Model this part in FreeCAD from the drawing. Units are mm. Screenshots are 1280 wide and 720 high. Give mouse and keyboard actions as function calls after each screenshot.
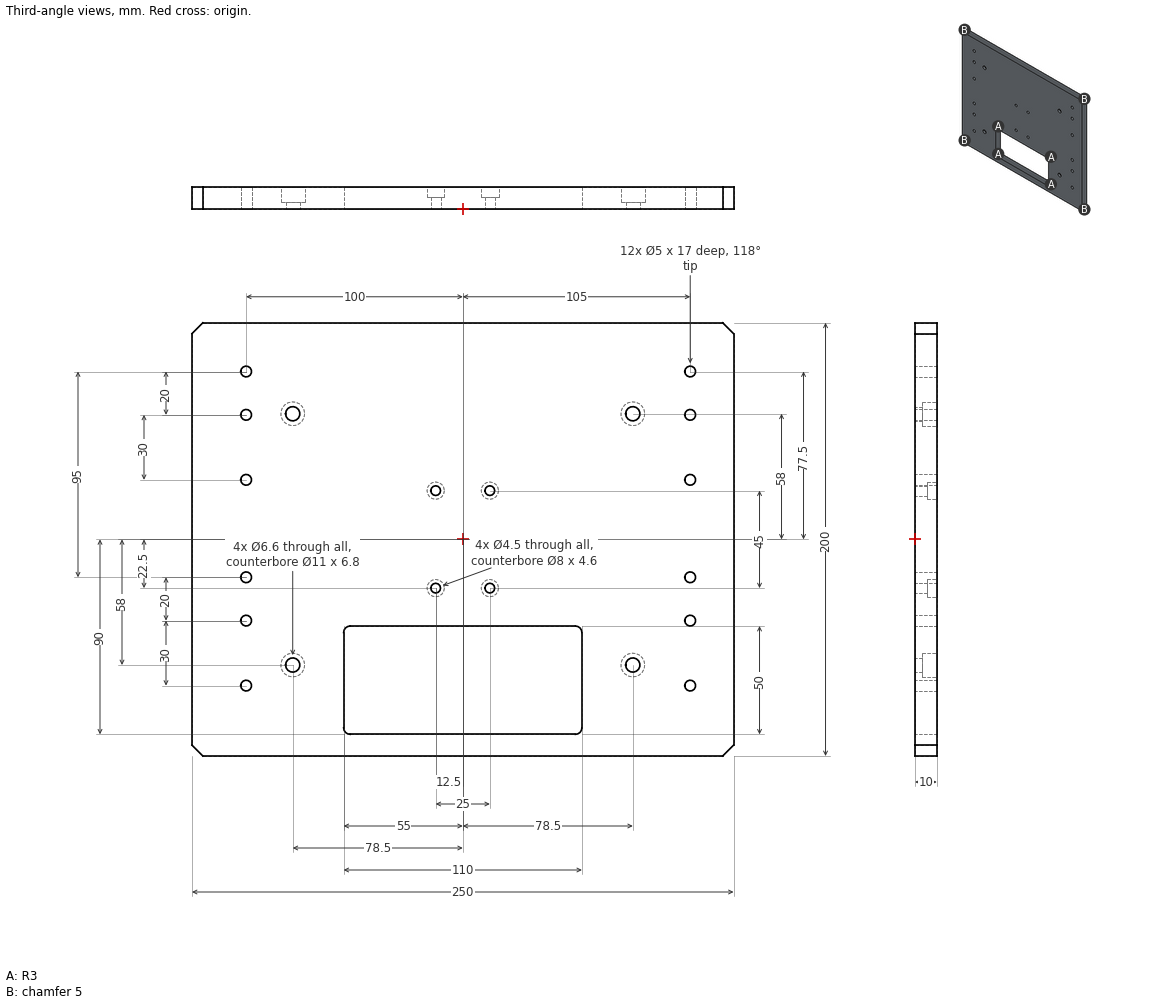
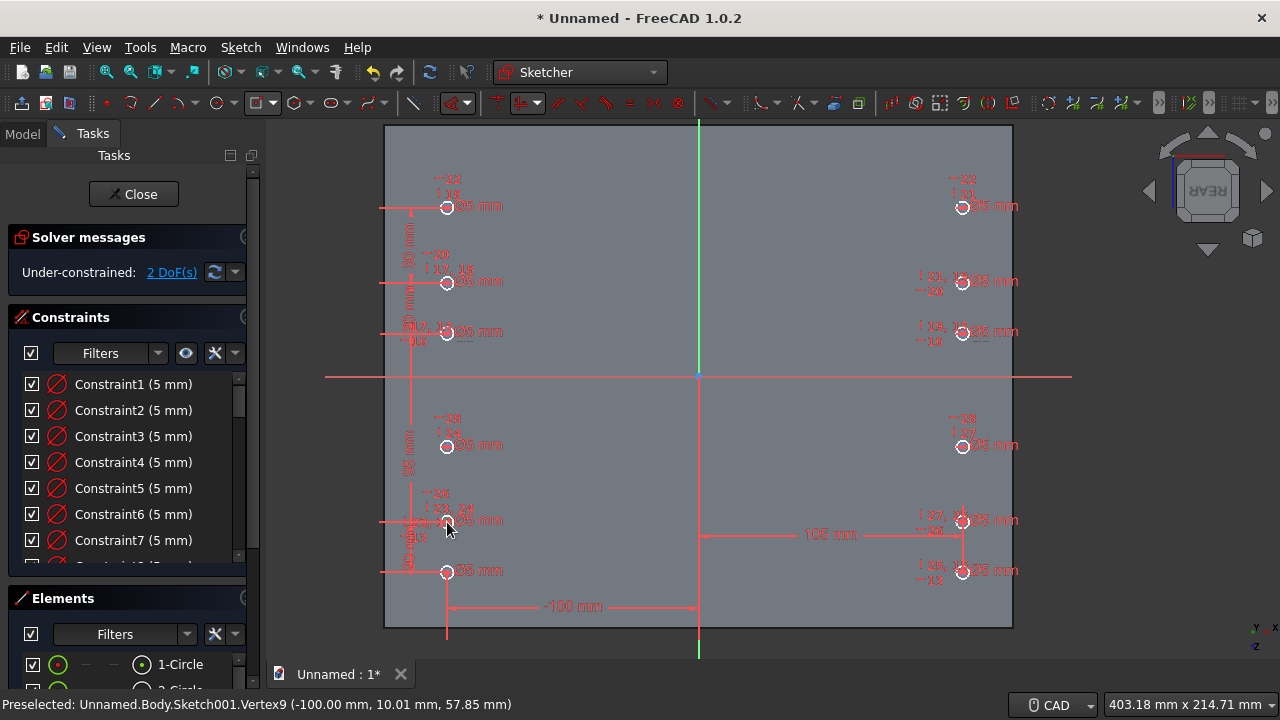
click(447, 447)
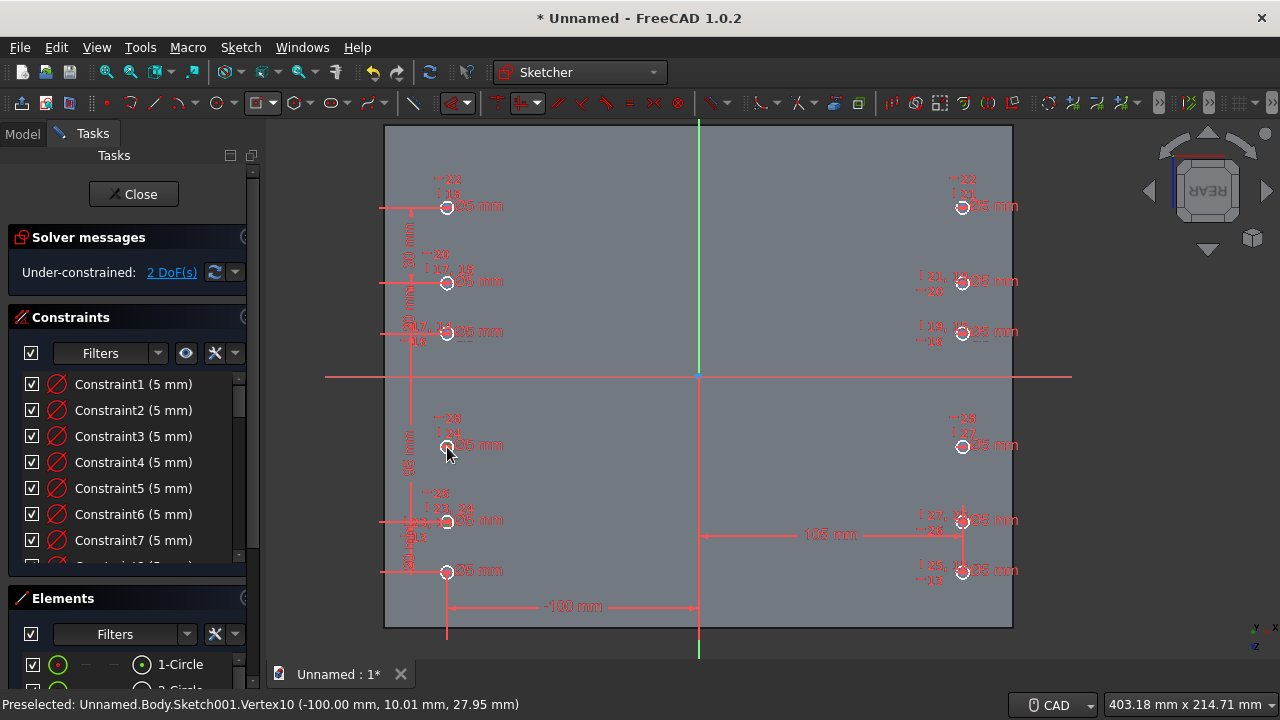
click(470, 104)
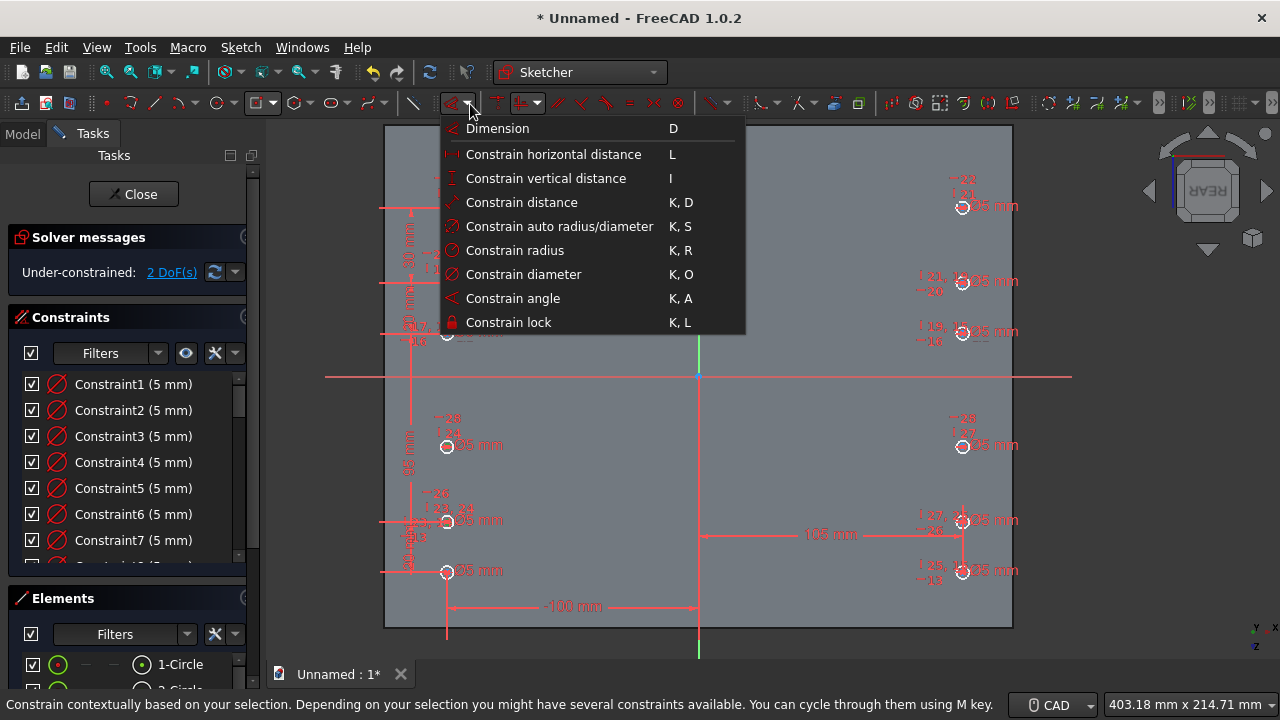
click(593, 178)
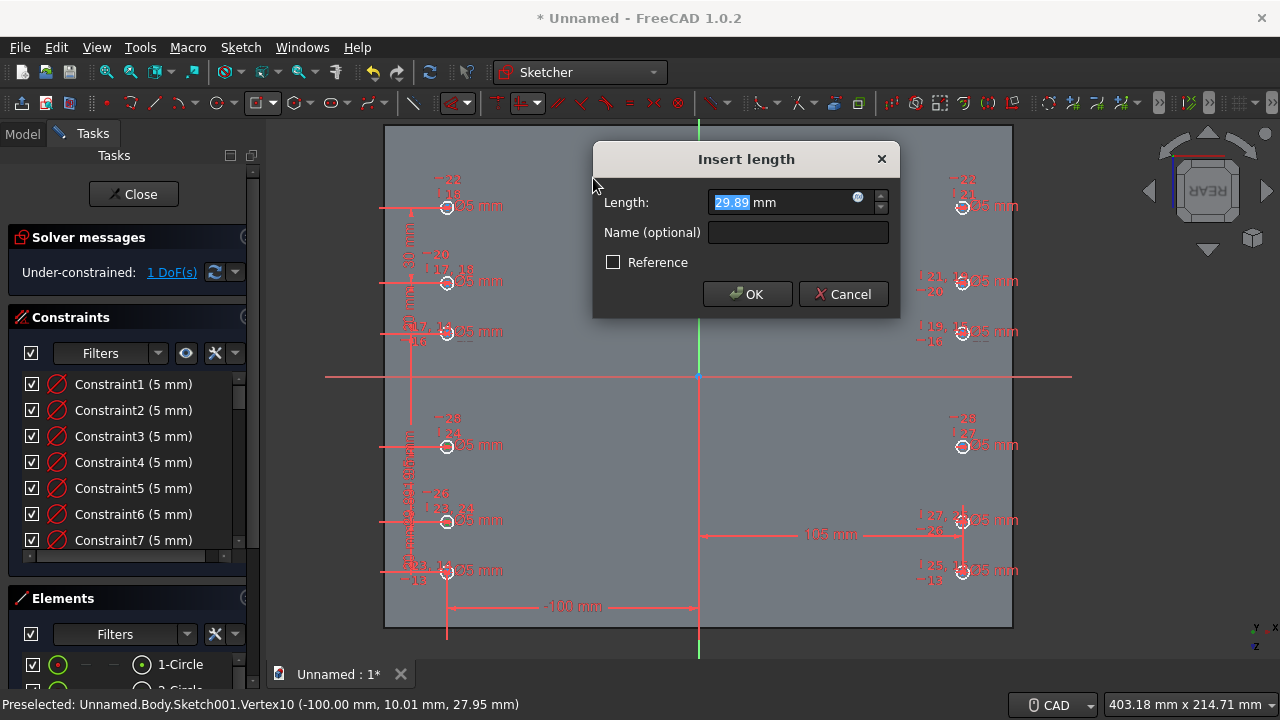
text(30)
key(Return)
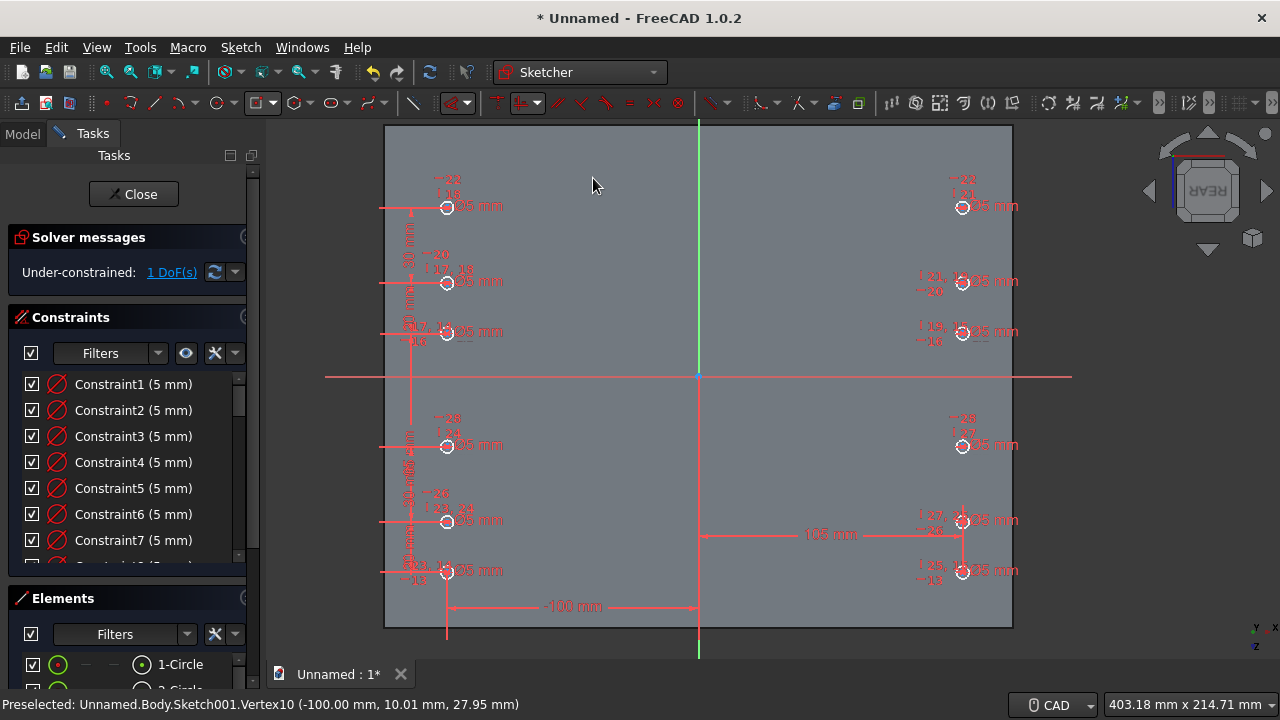
click(963, 572)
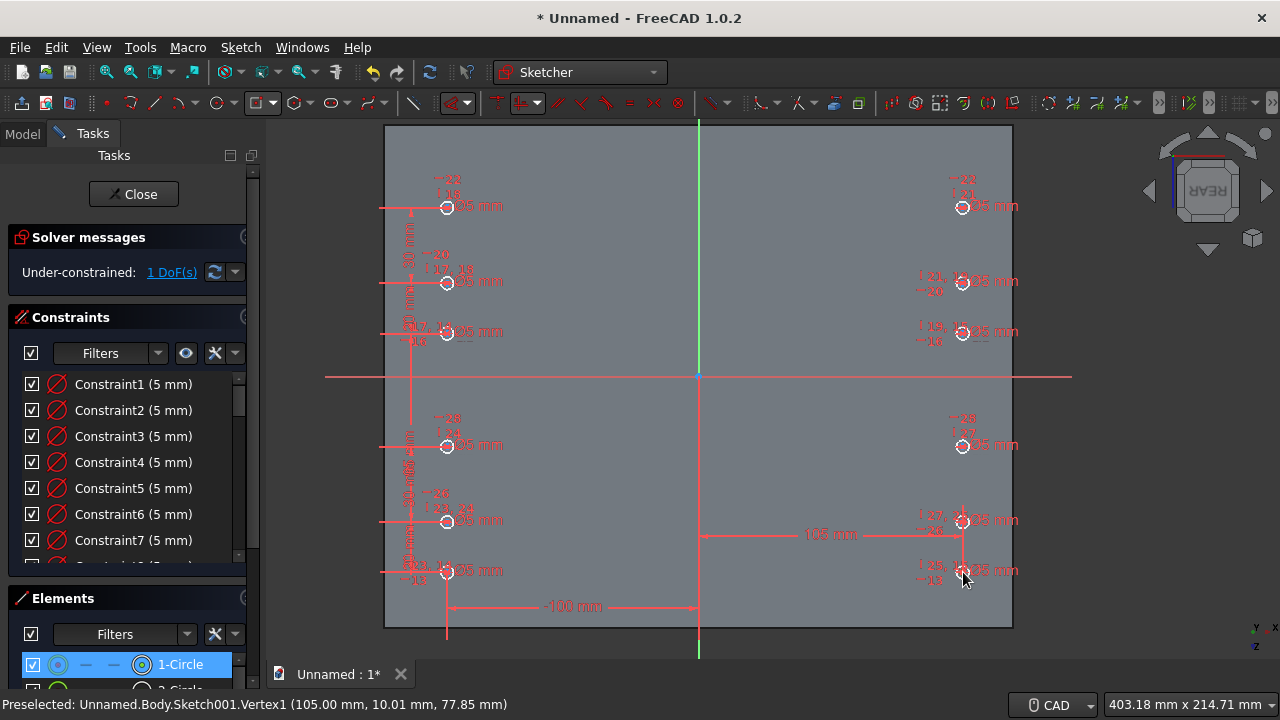
key(i)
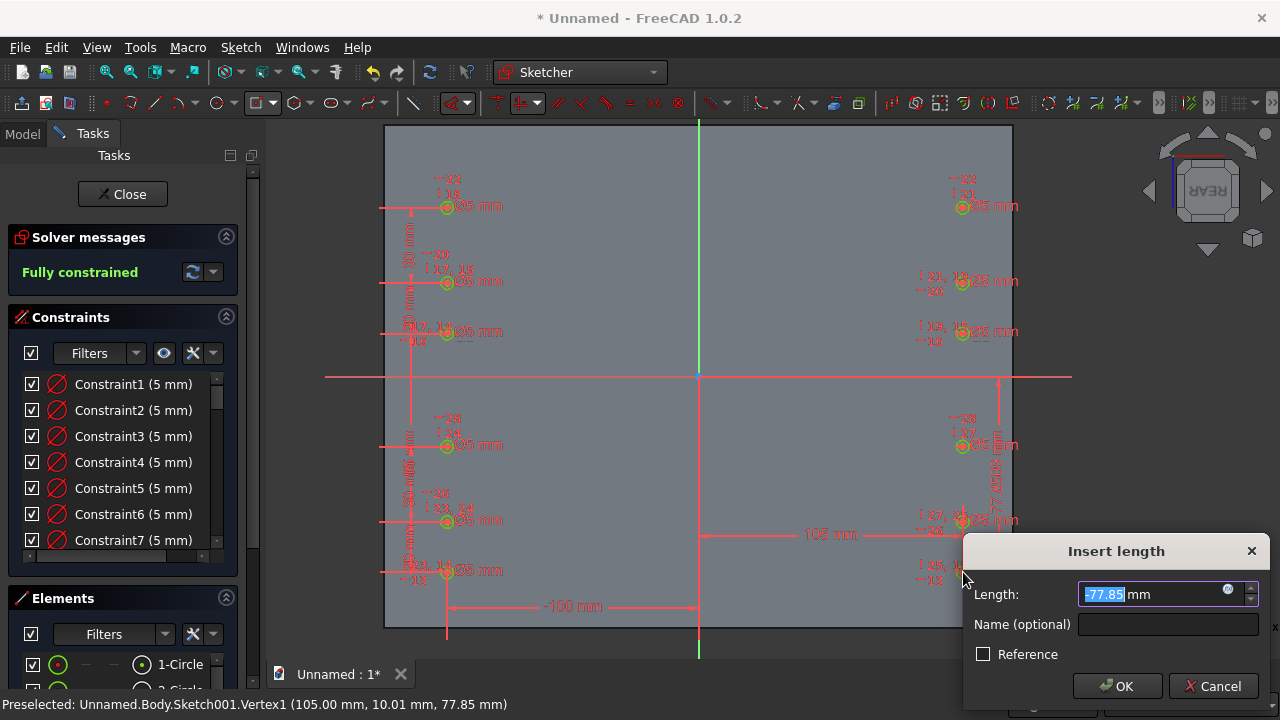
text(-77.5)
key(Return)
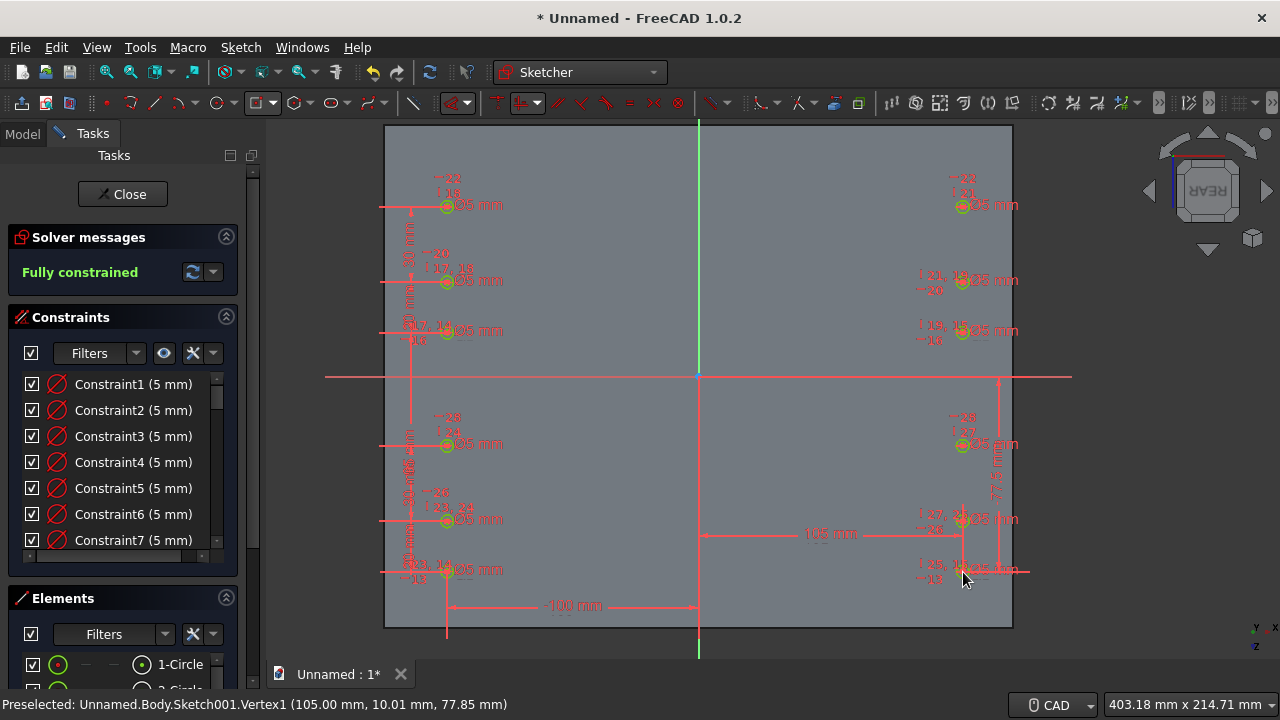
click(123, 194)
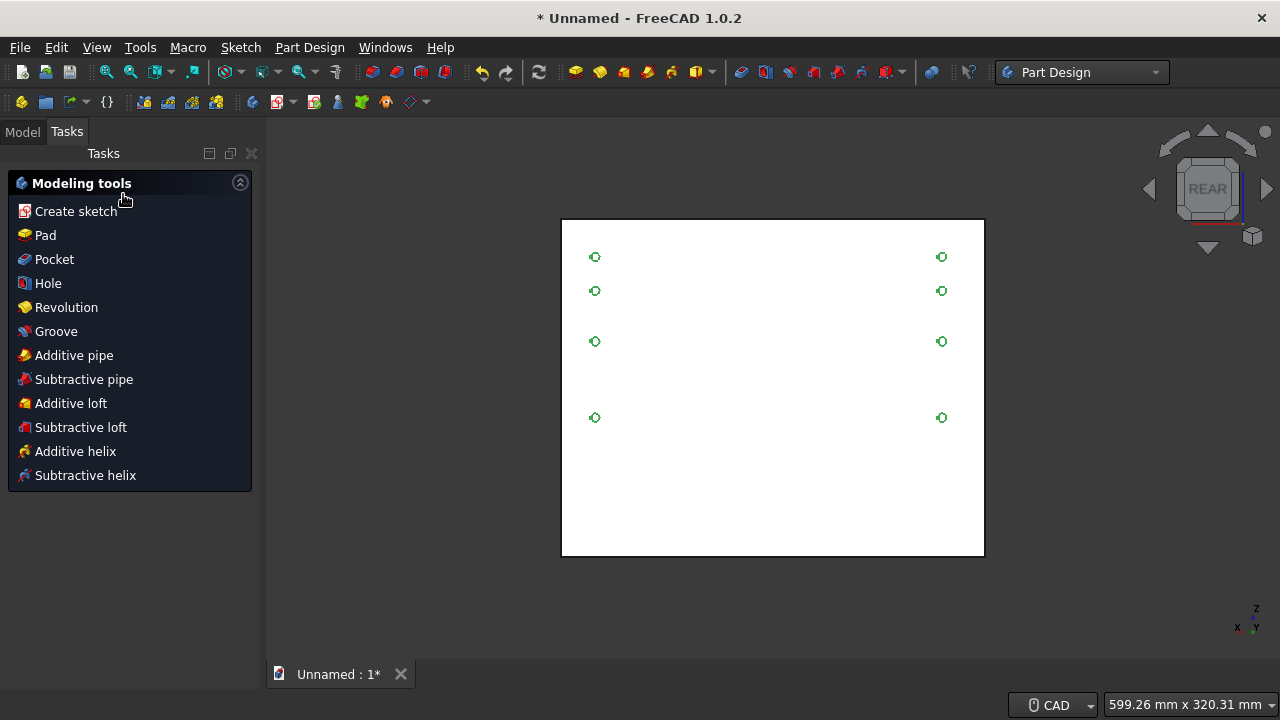
click(766, 72)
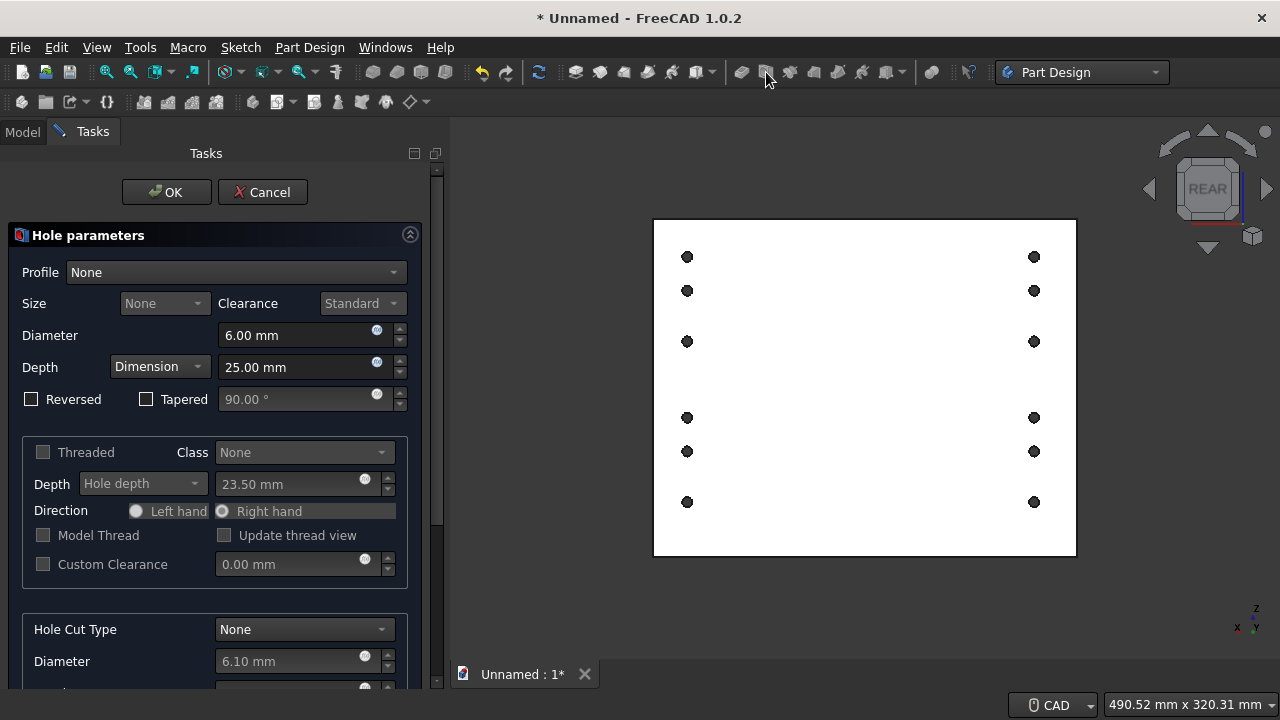
triple_click(305, 335)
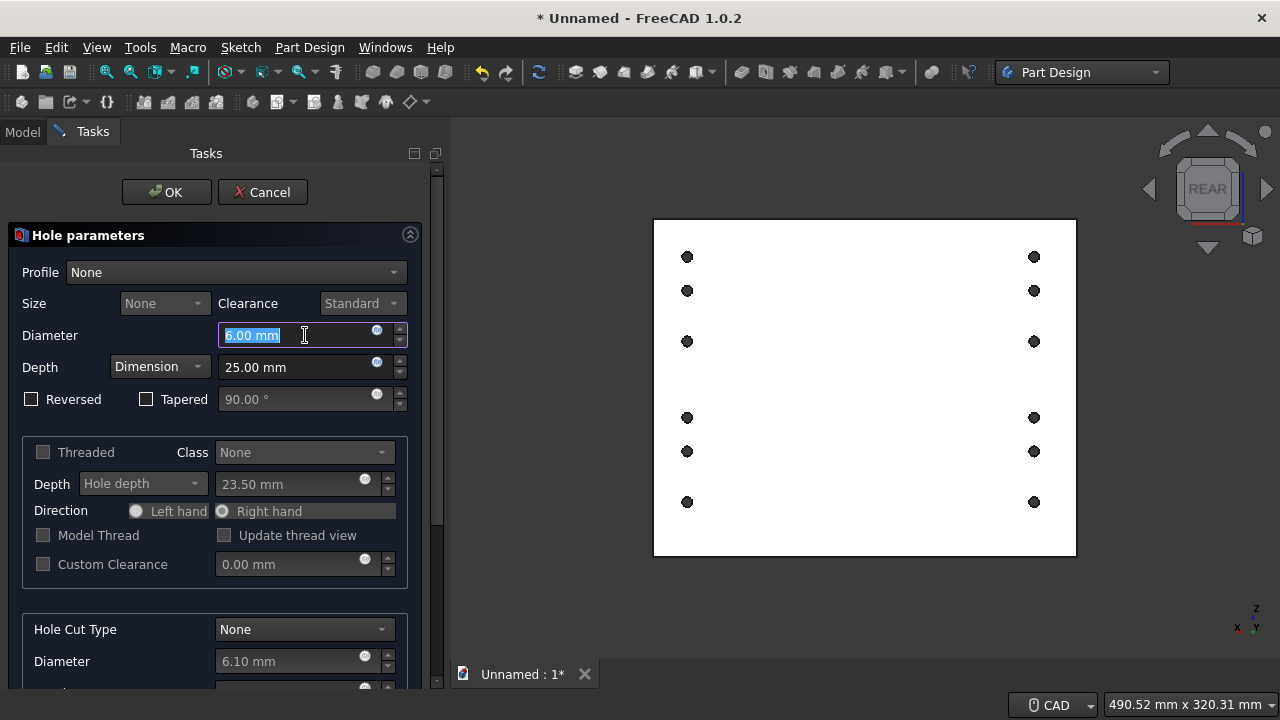
text(5)
key(Tab)